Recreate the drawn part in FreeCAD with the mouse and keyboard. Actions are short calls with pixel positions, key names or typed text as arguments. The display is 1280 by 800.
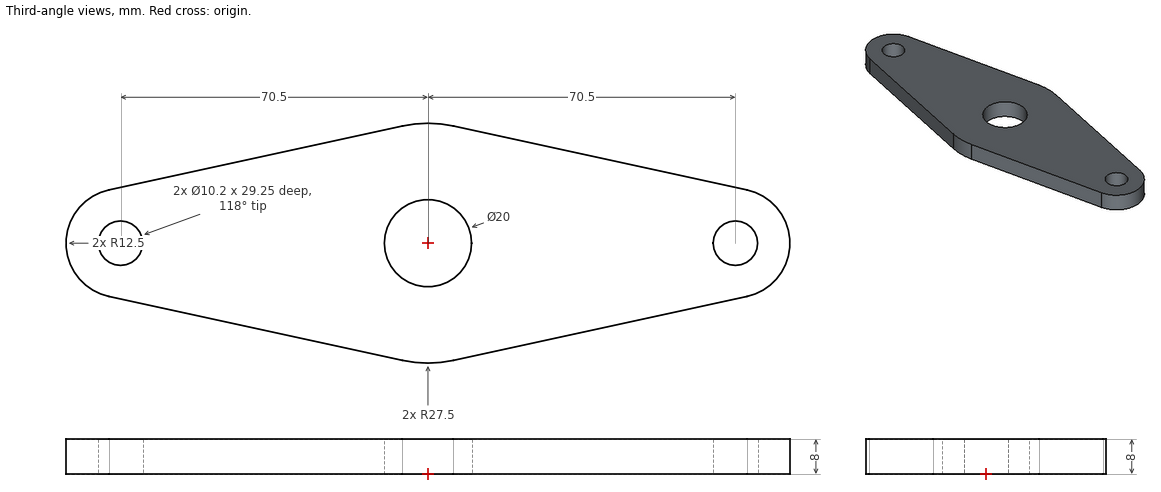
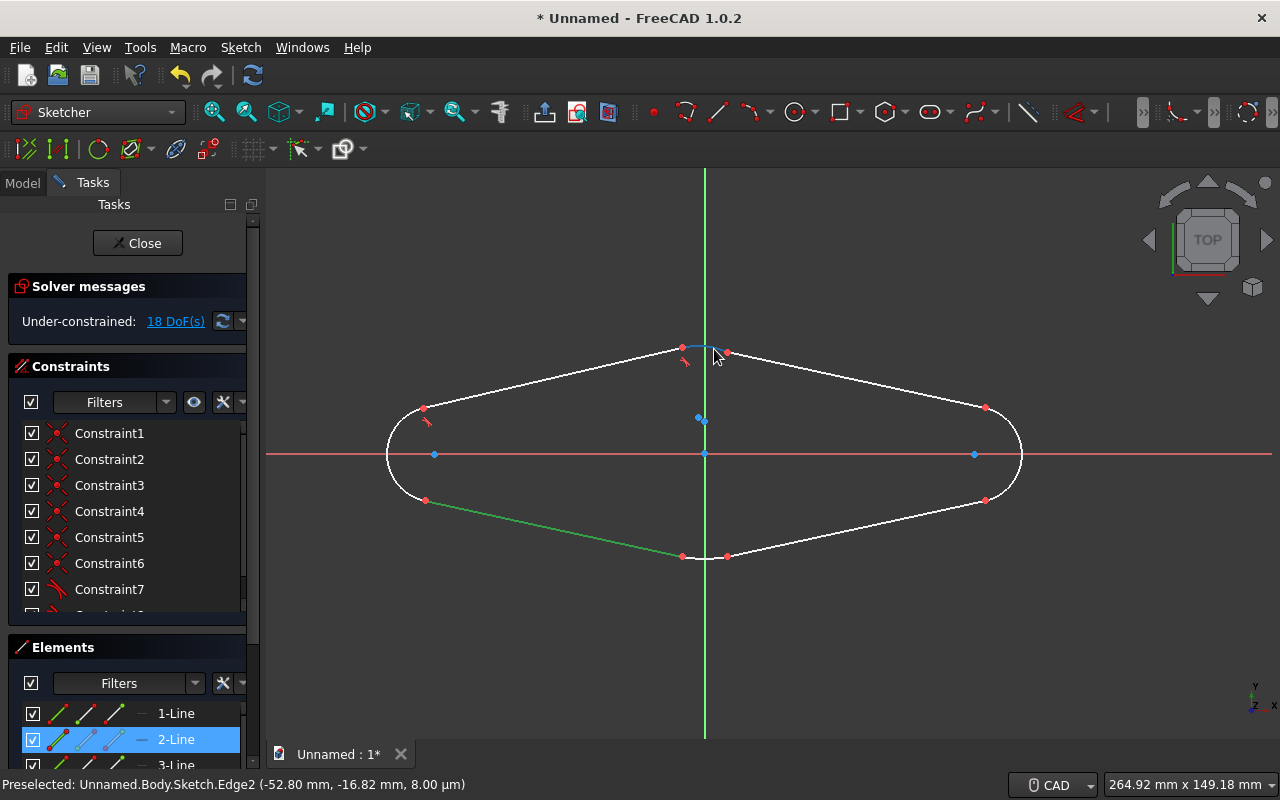
click(394, 430)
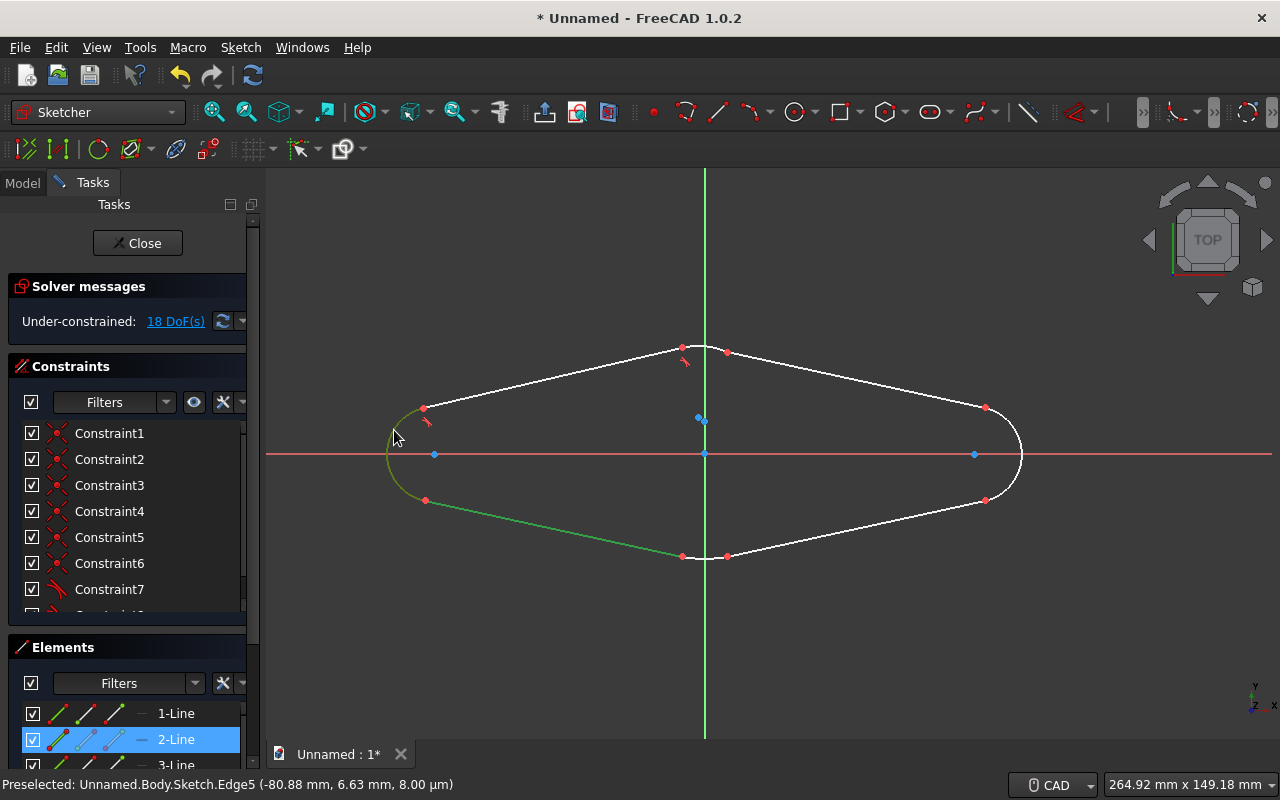
key(t)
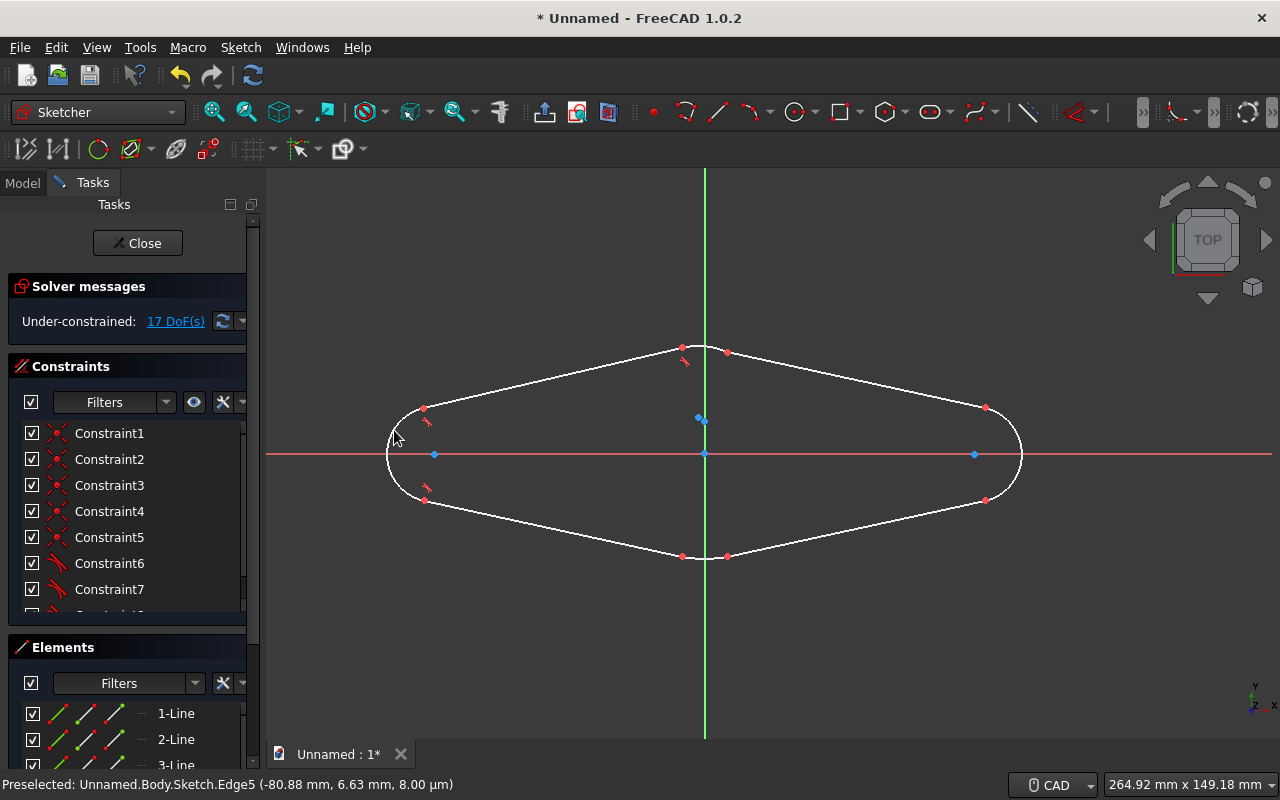
click(502, 518)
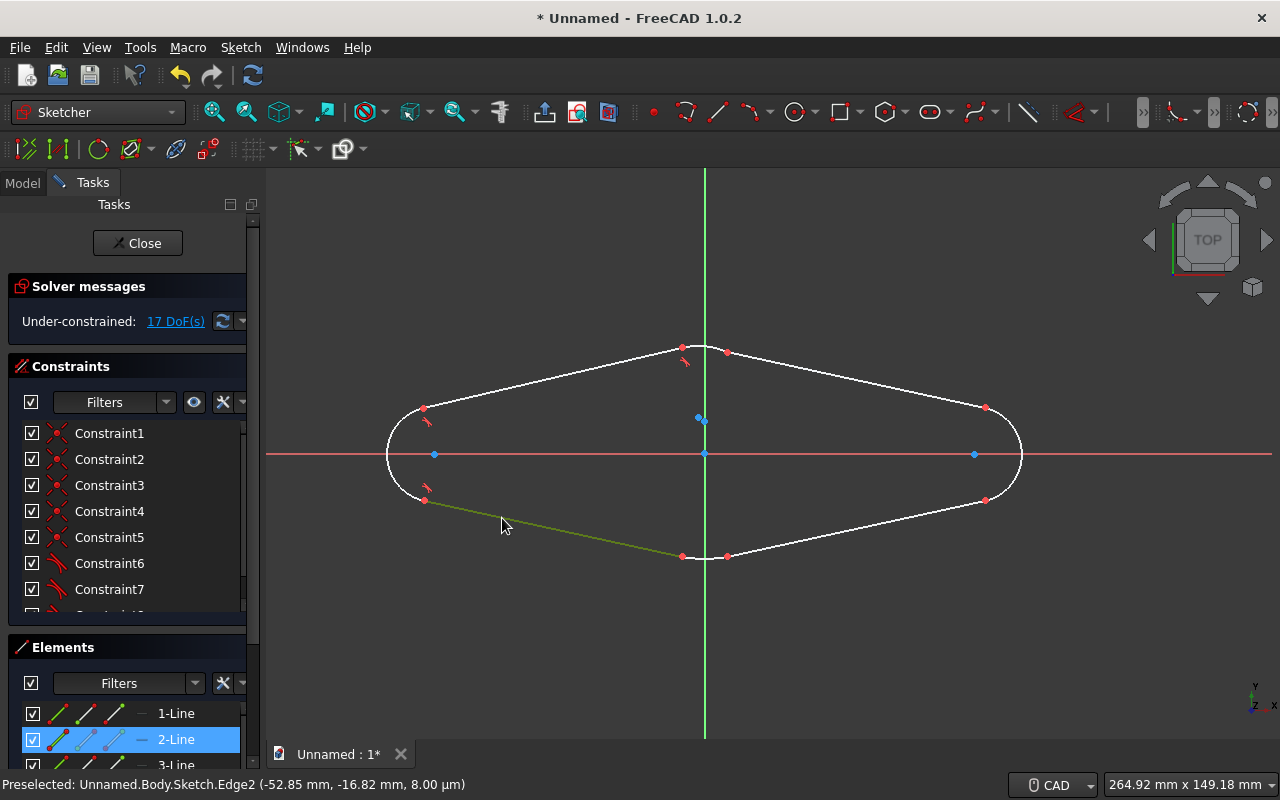
scroll(695, 559, up, 3)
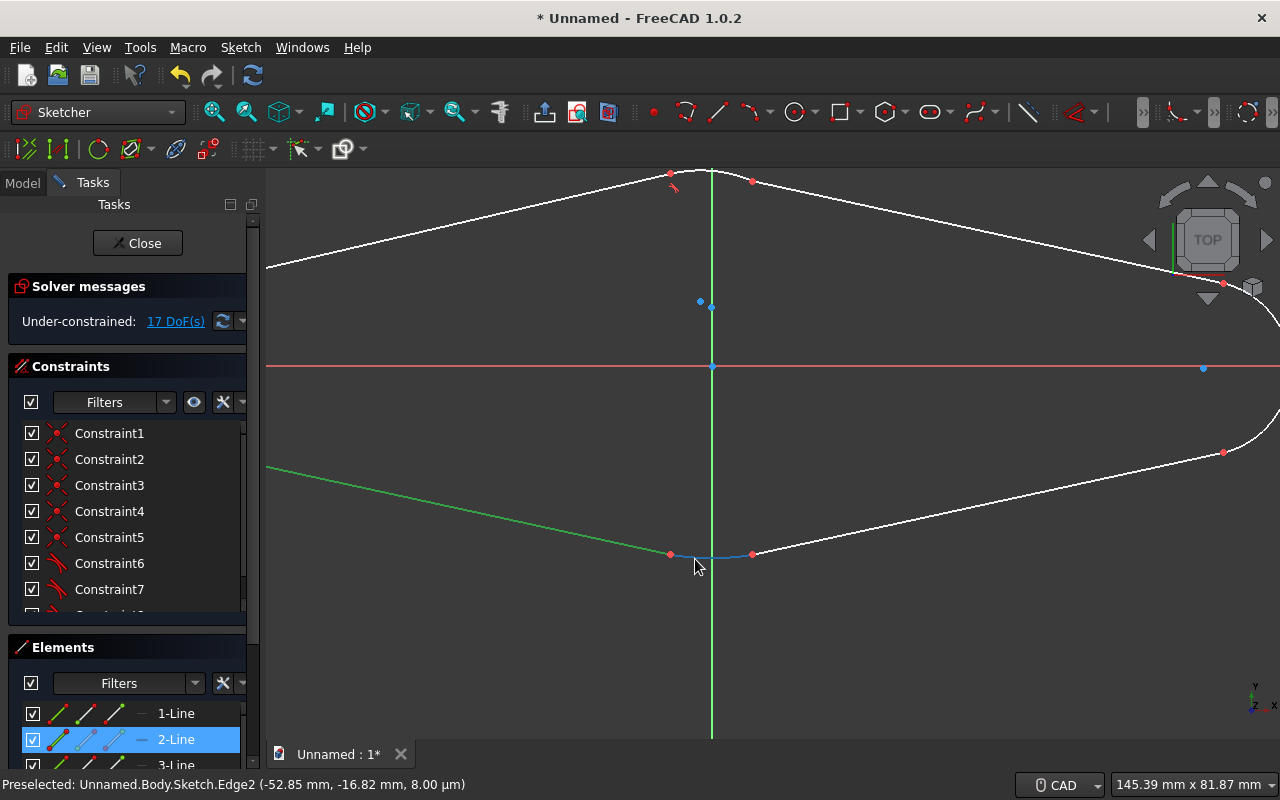
click(696, 558)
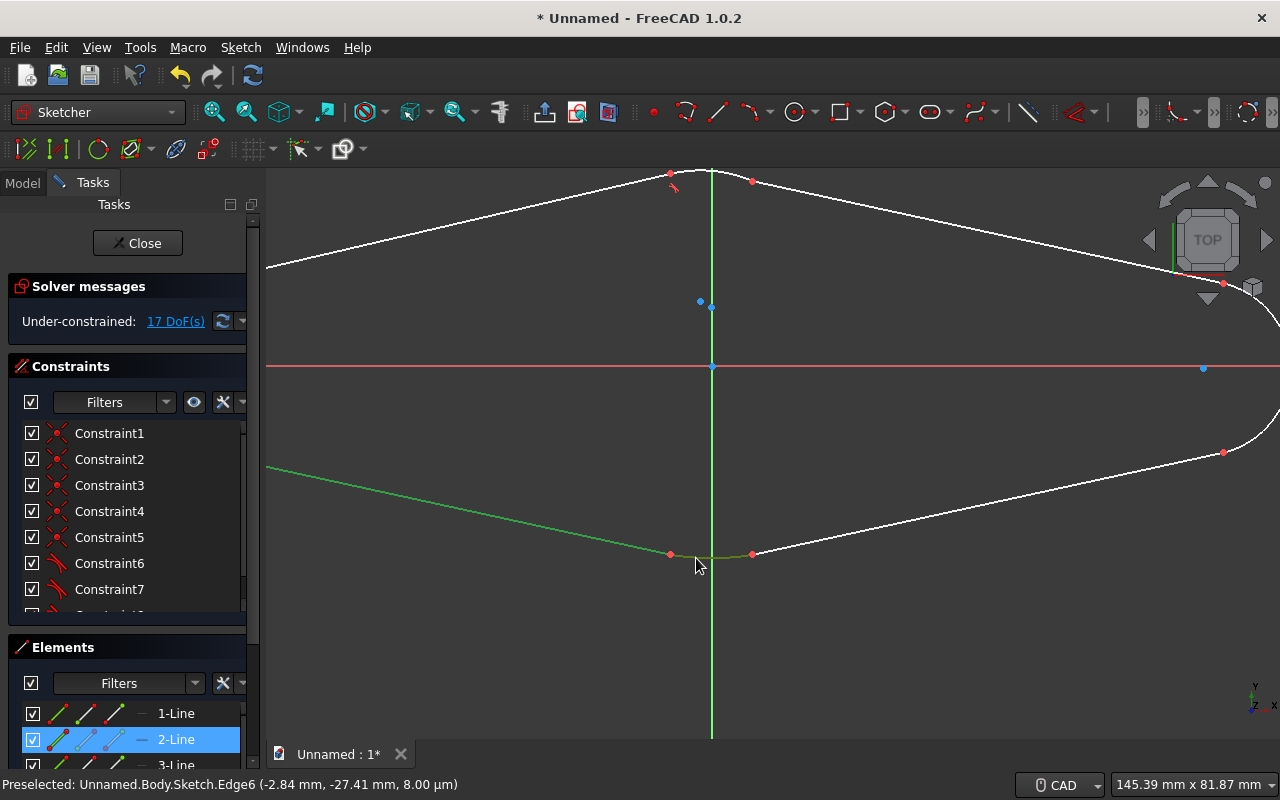
key(t)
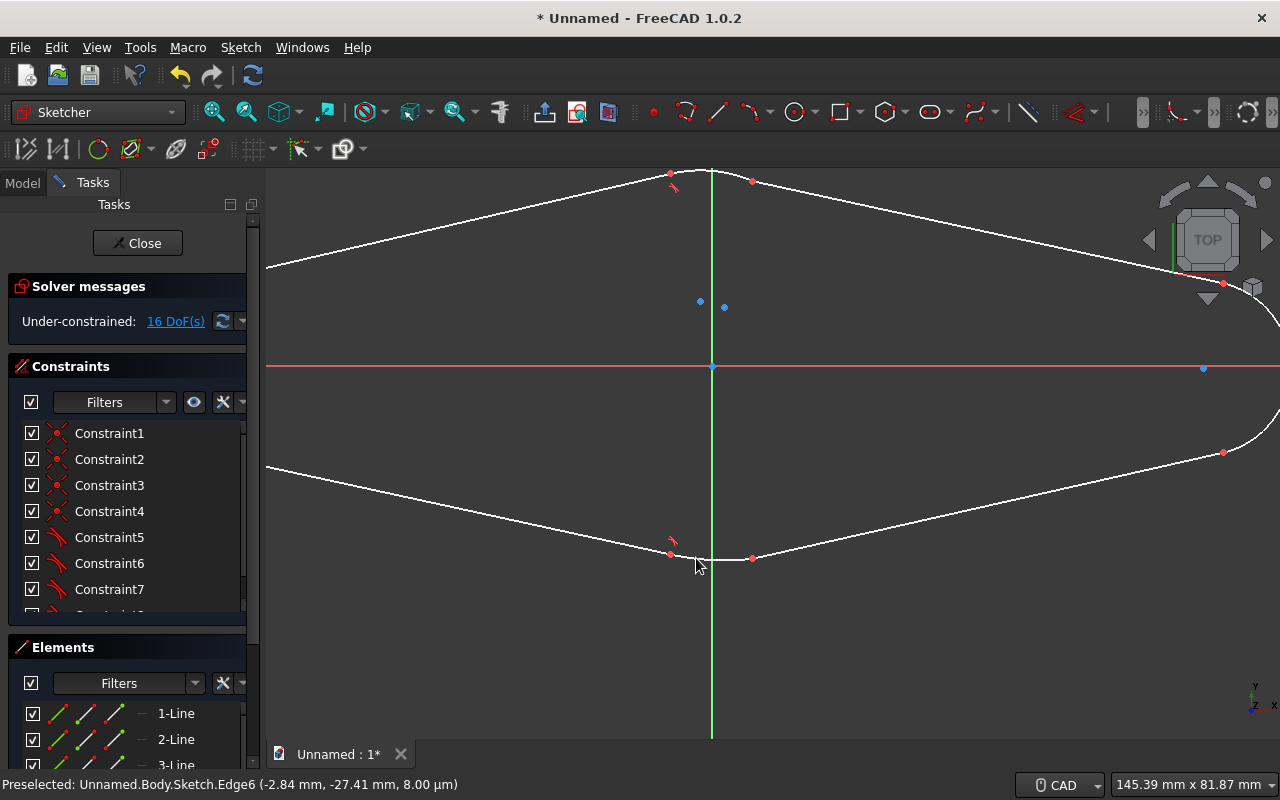
click(894, 527)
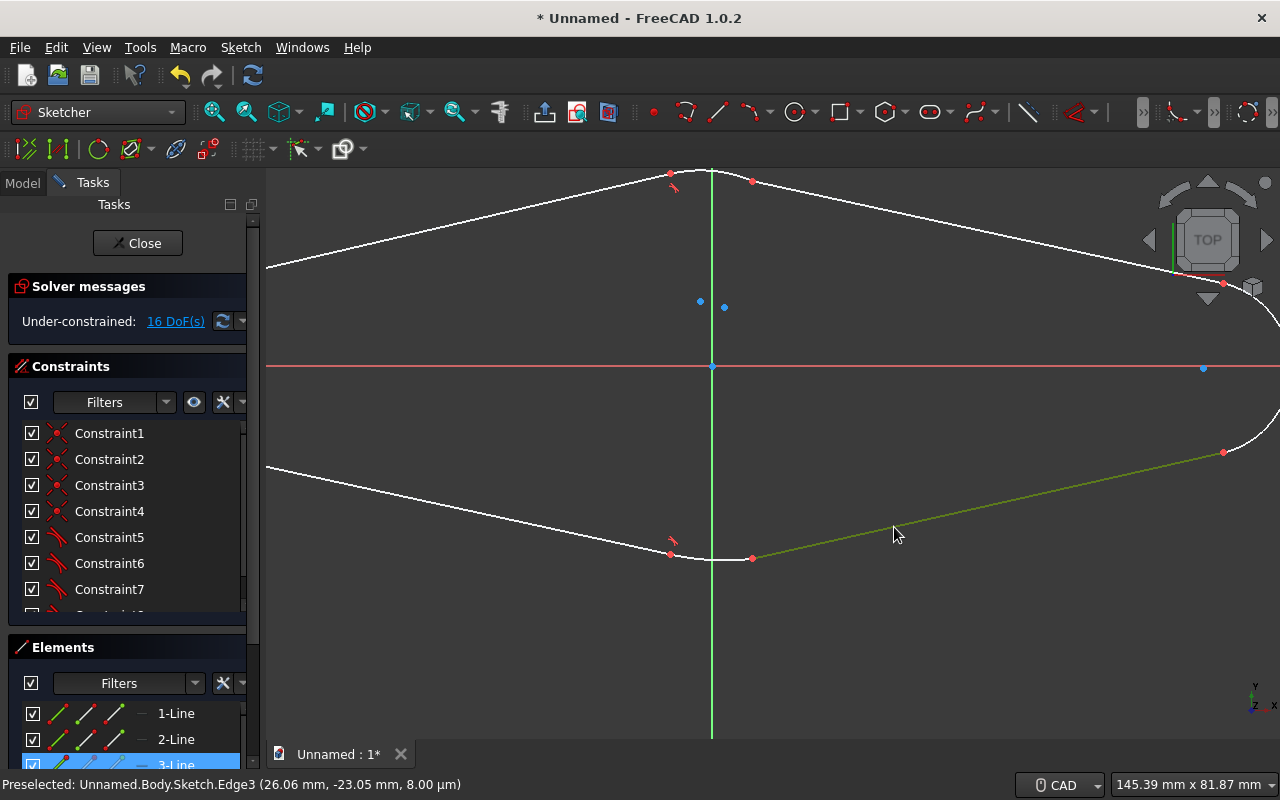
click(695, 559)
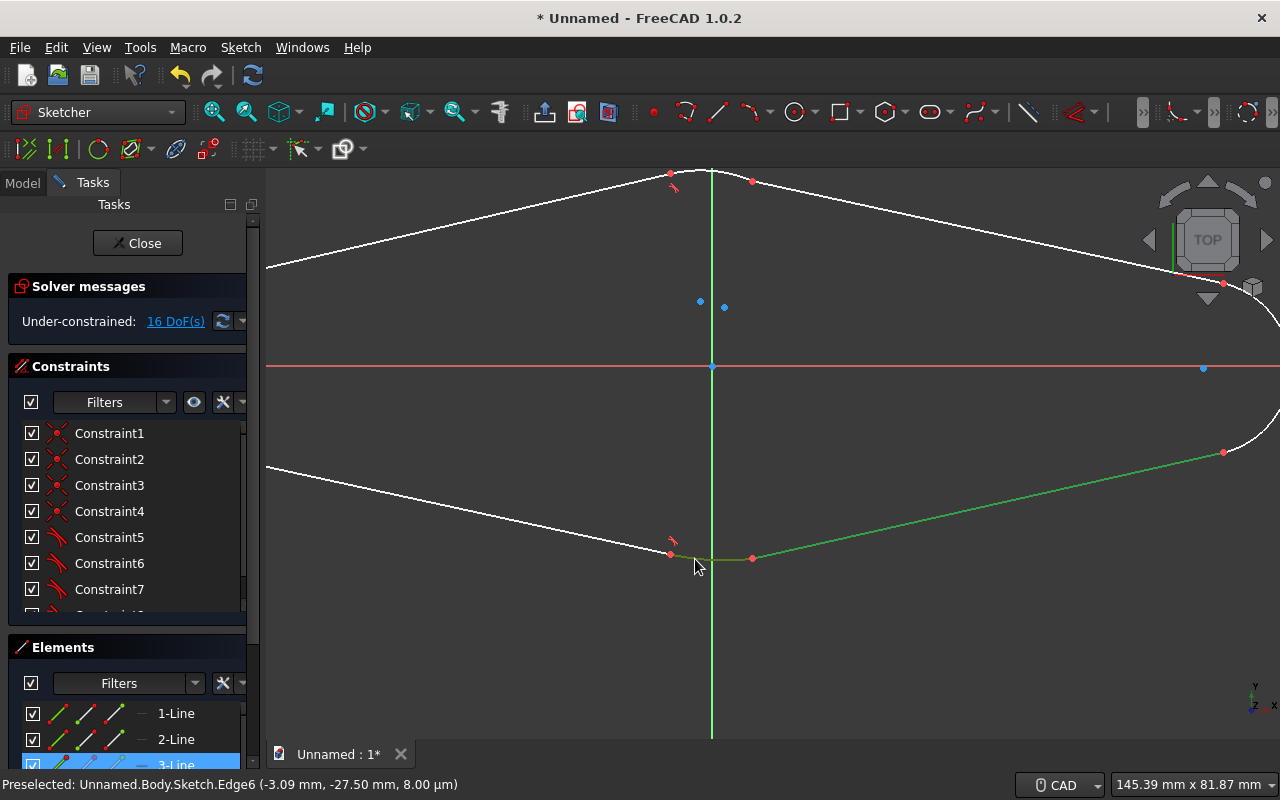
key(t)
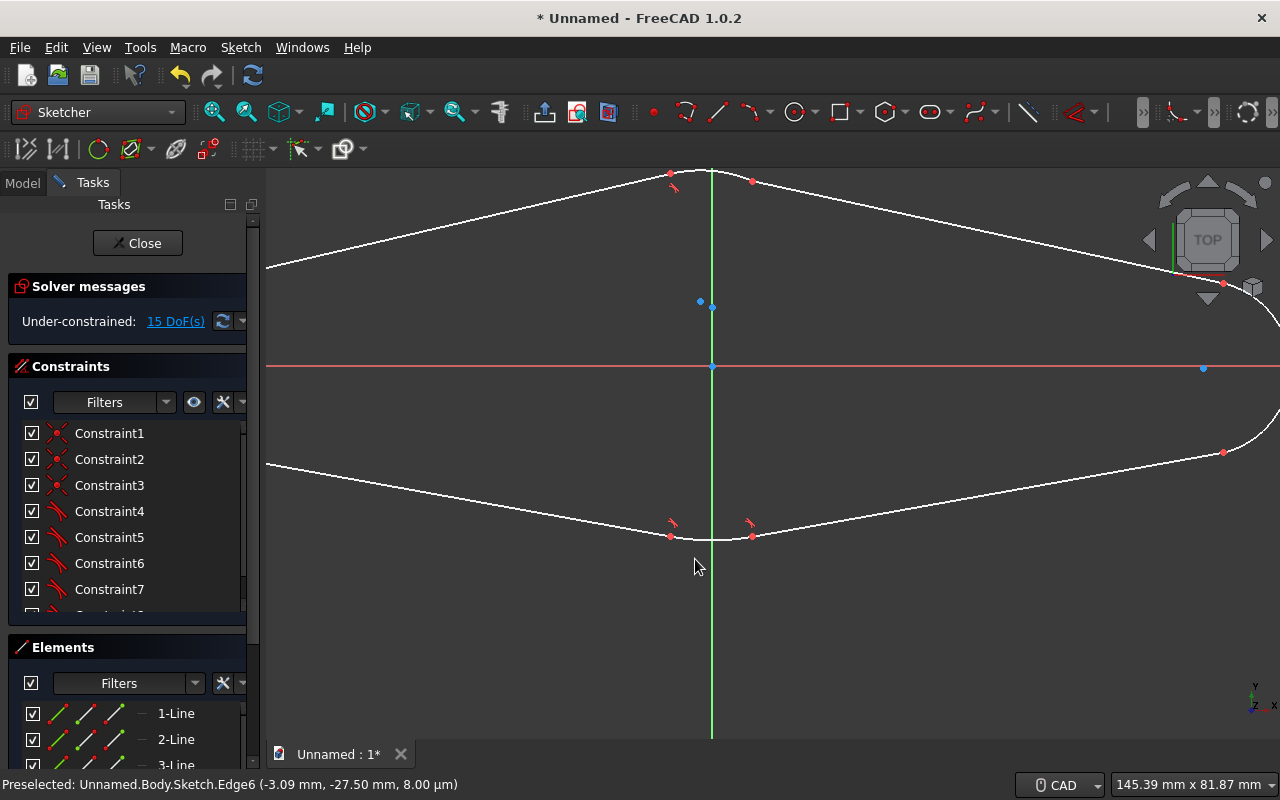
click(894, 512)